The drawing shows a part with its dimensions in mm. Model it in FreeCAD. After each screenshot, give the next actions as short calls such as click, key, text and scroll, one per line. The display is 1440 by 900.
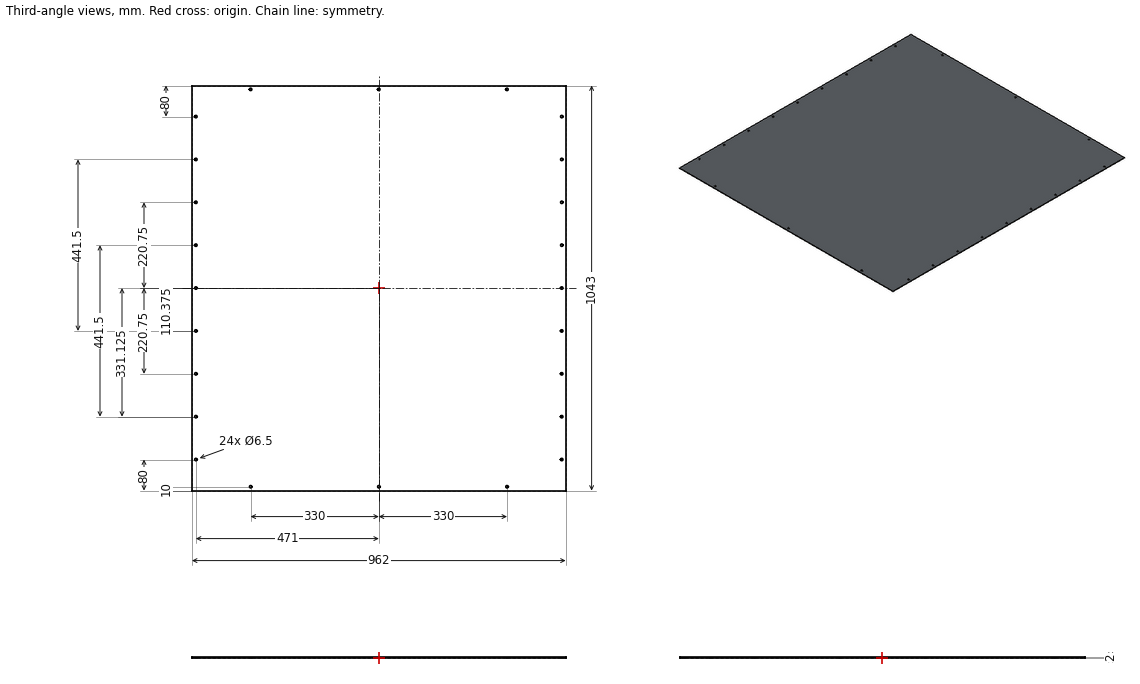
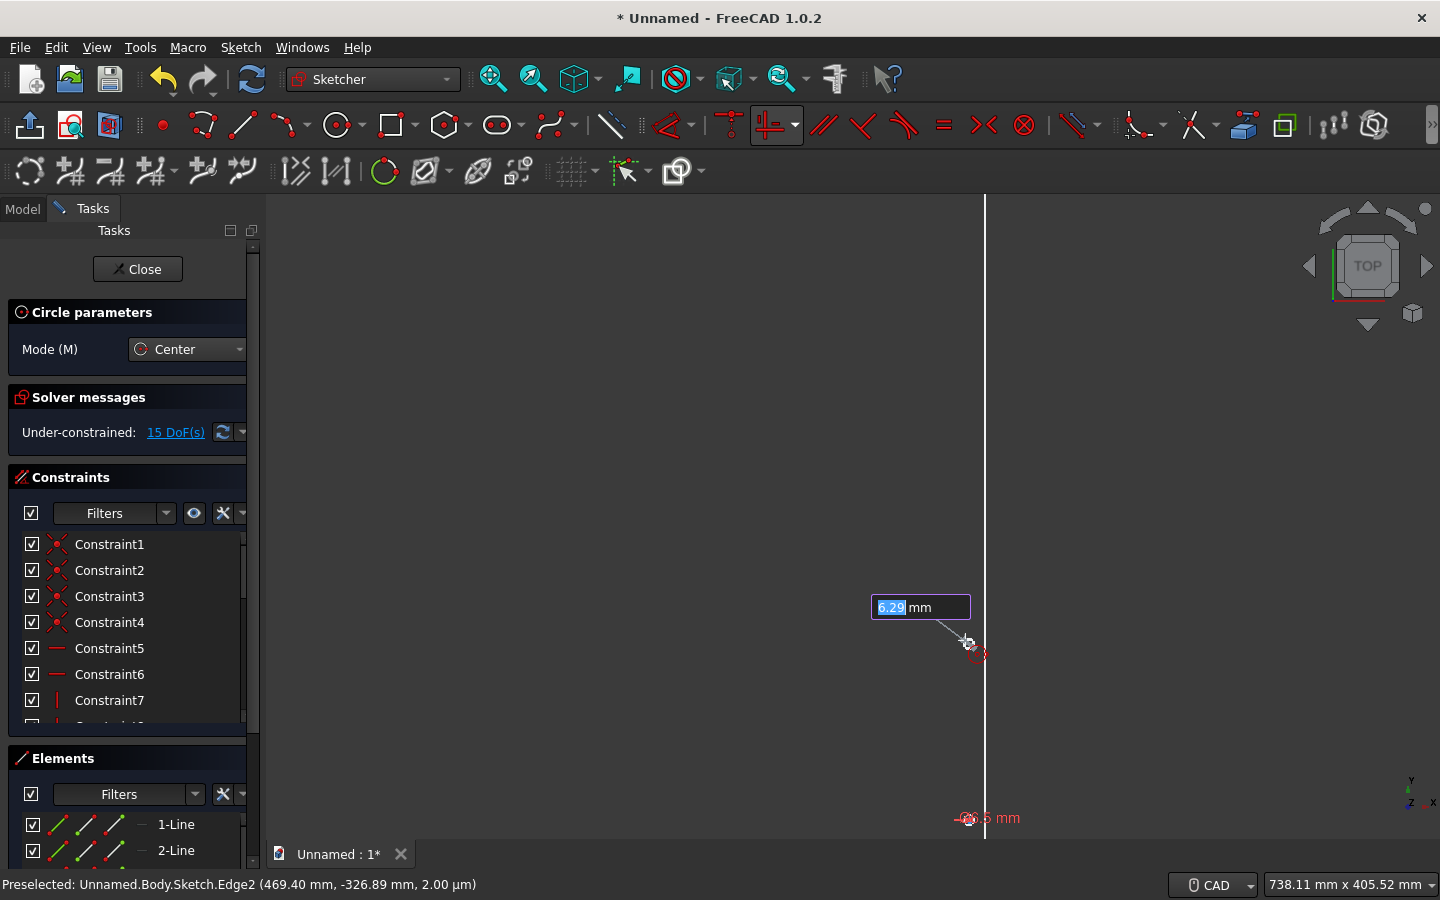
text(6.5)
key(Return)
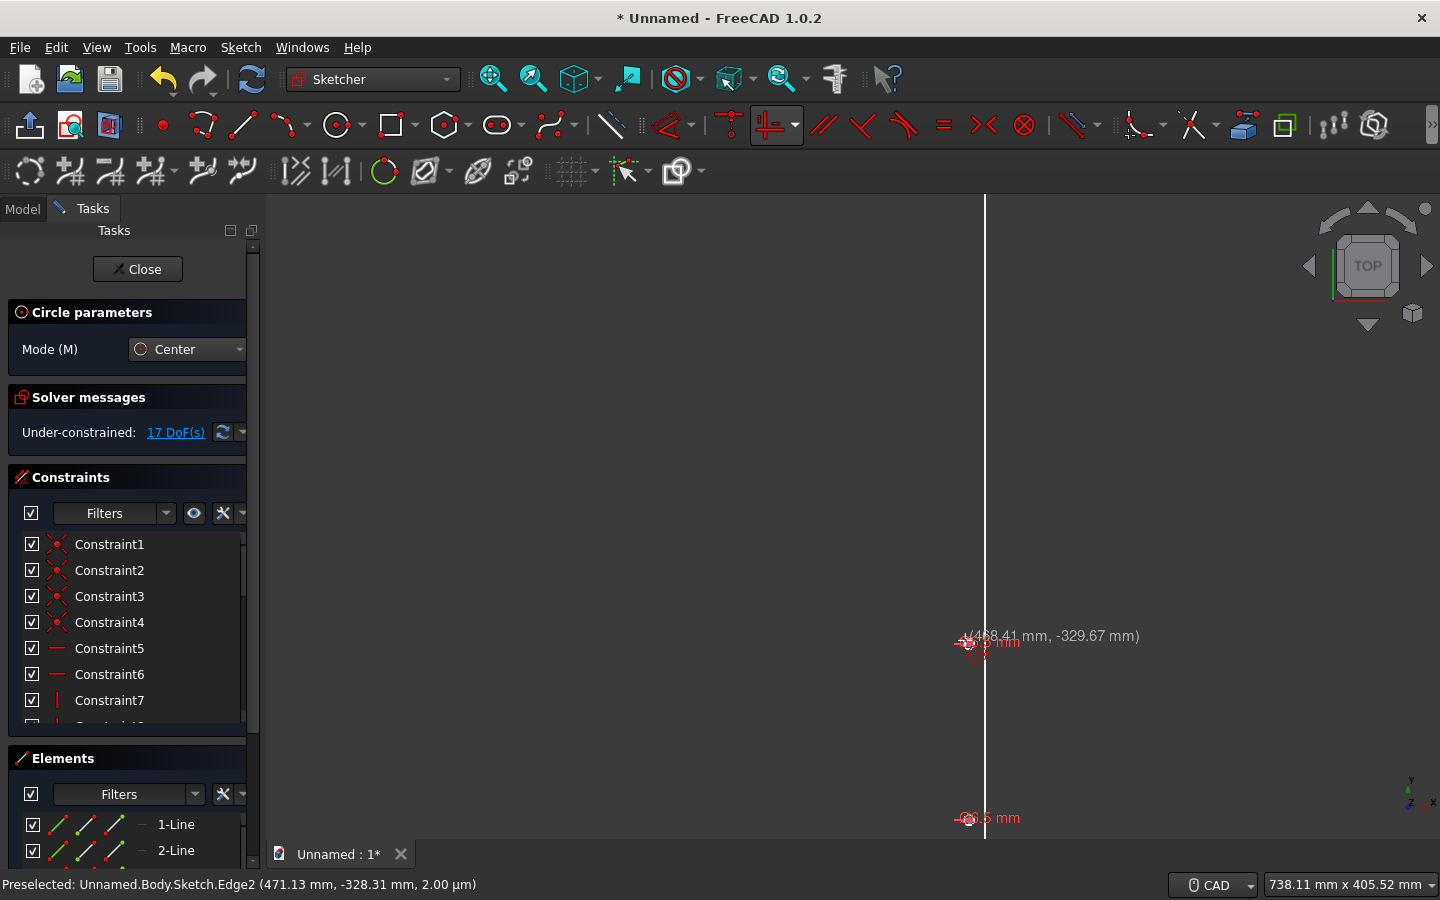
scroll(969, 468, up, 8)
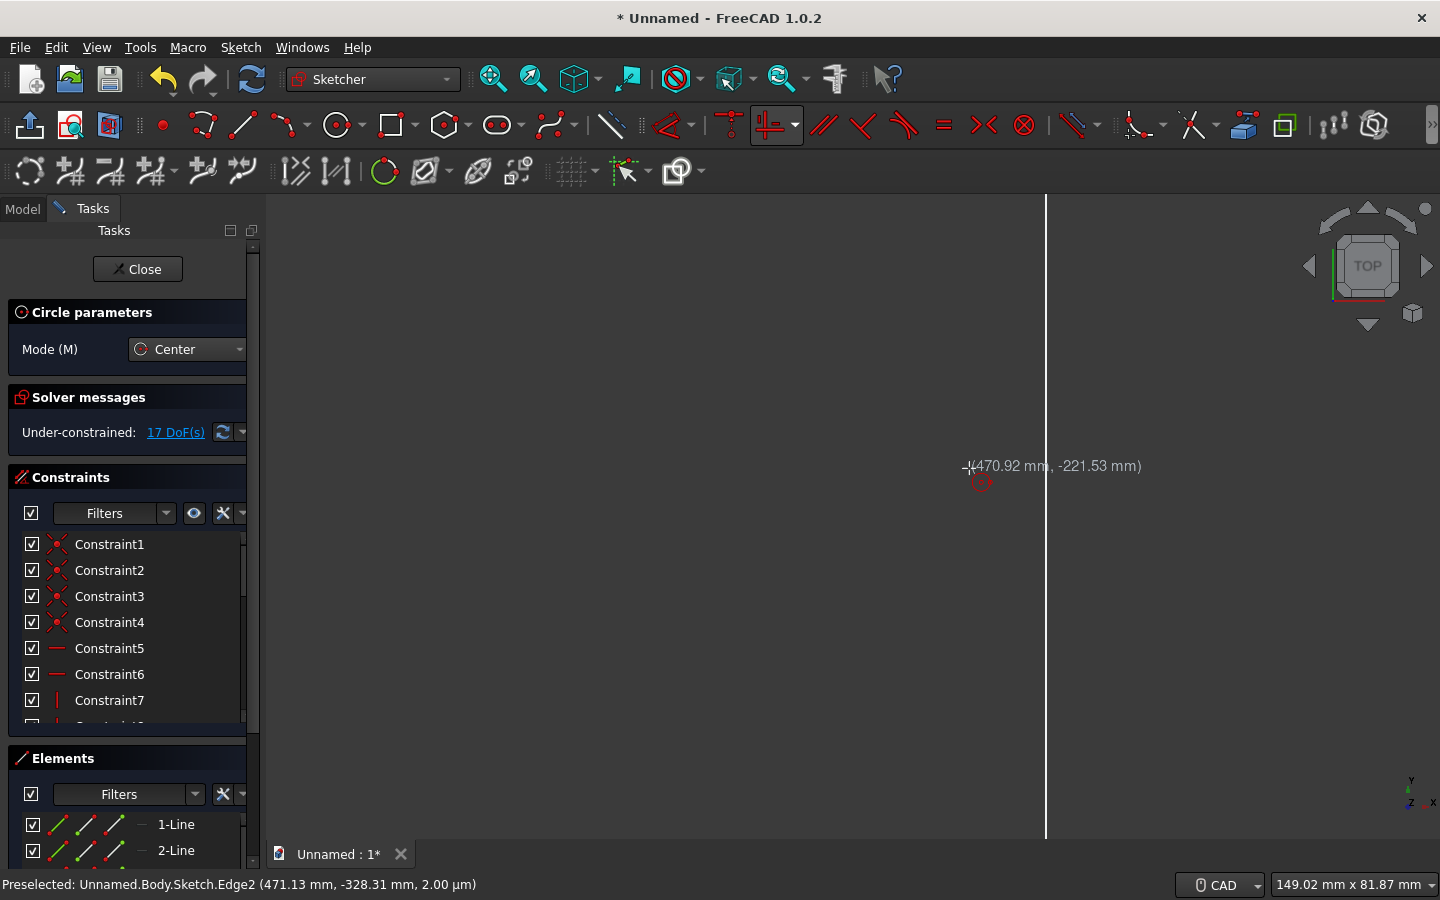
scroll(969, 610, down, 15)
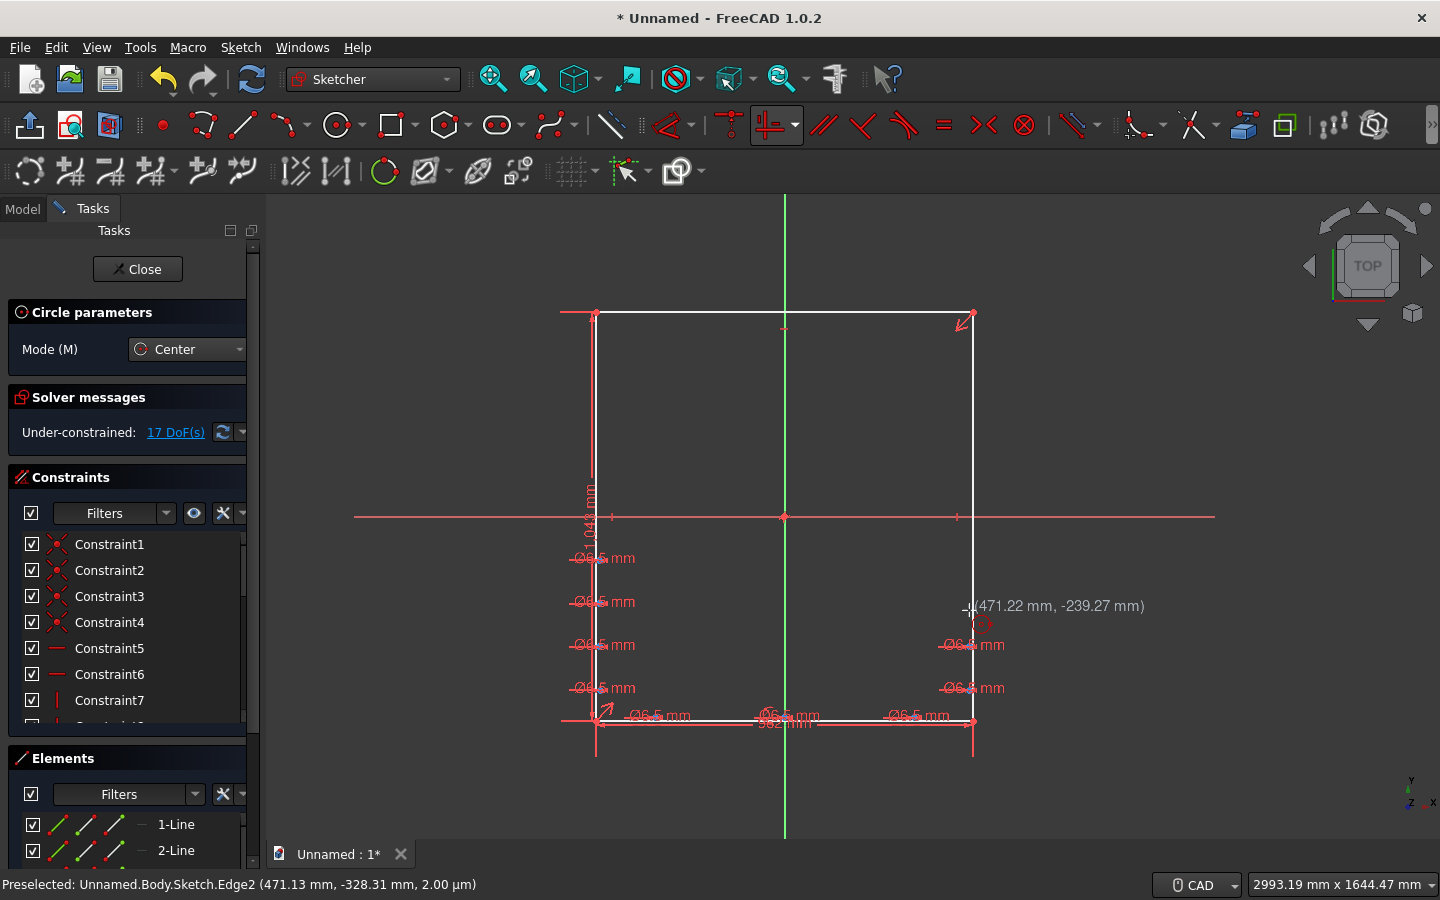
scroll(969, 603, up, 7)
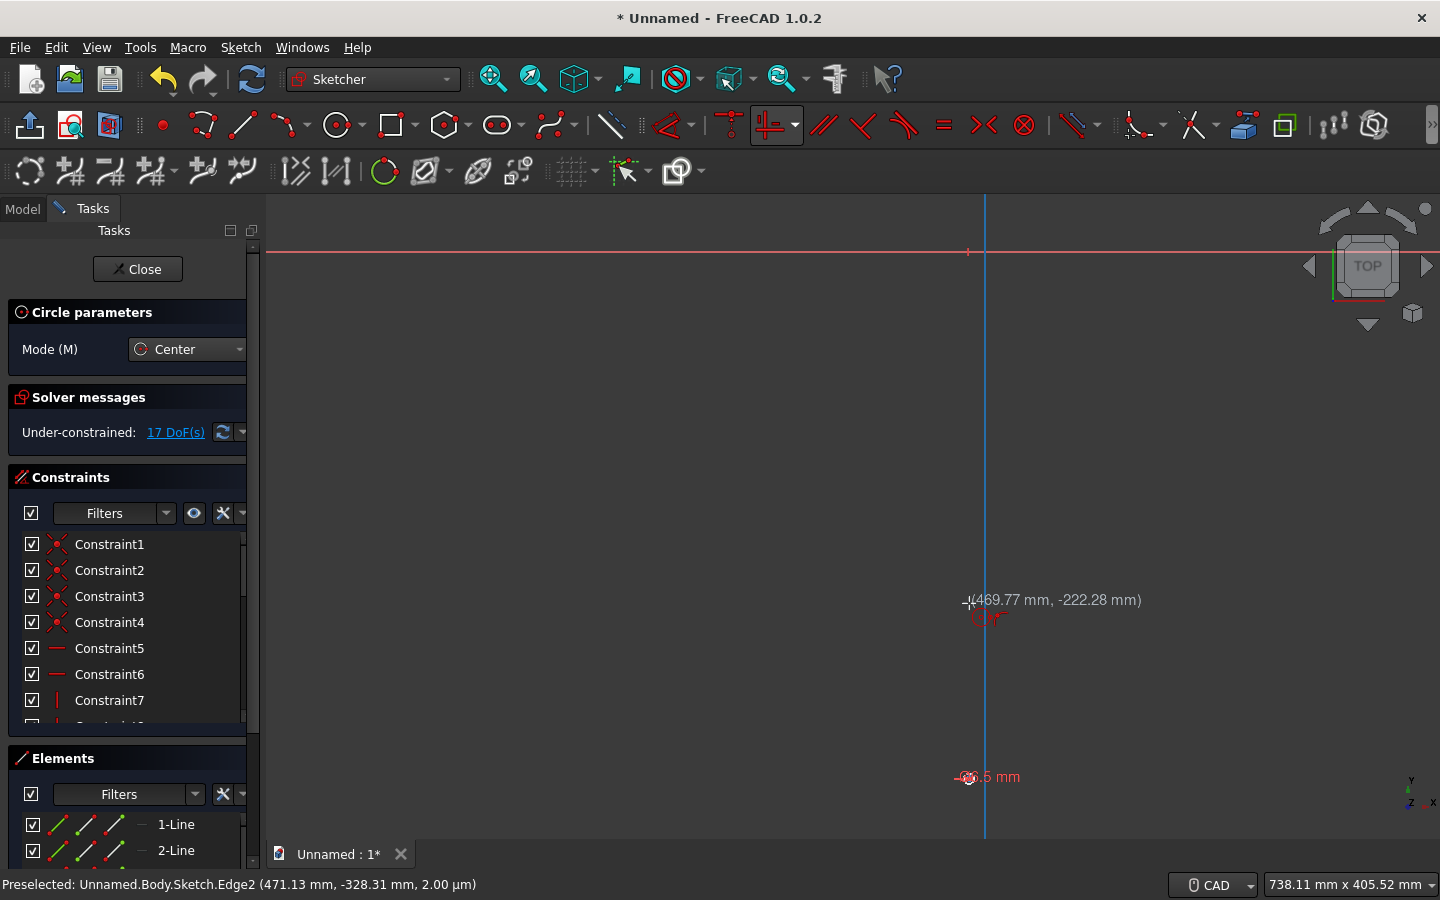
click(969, 603)
move(965, 599)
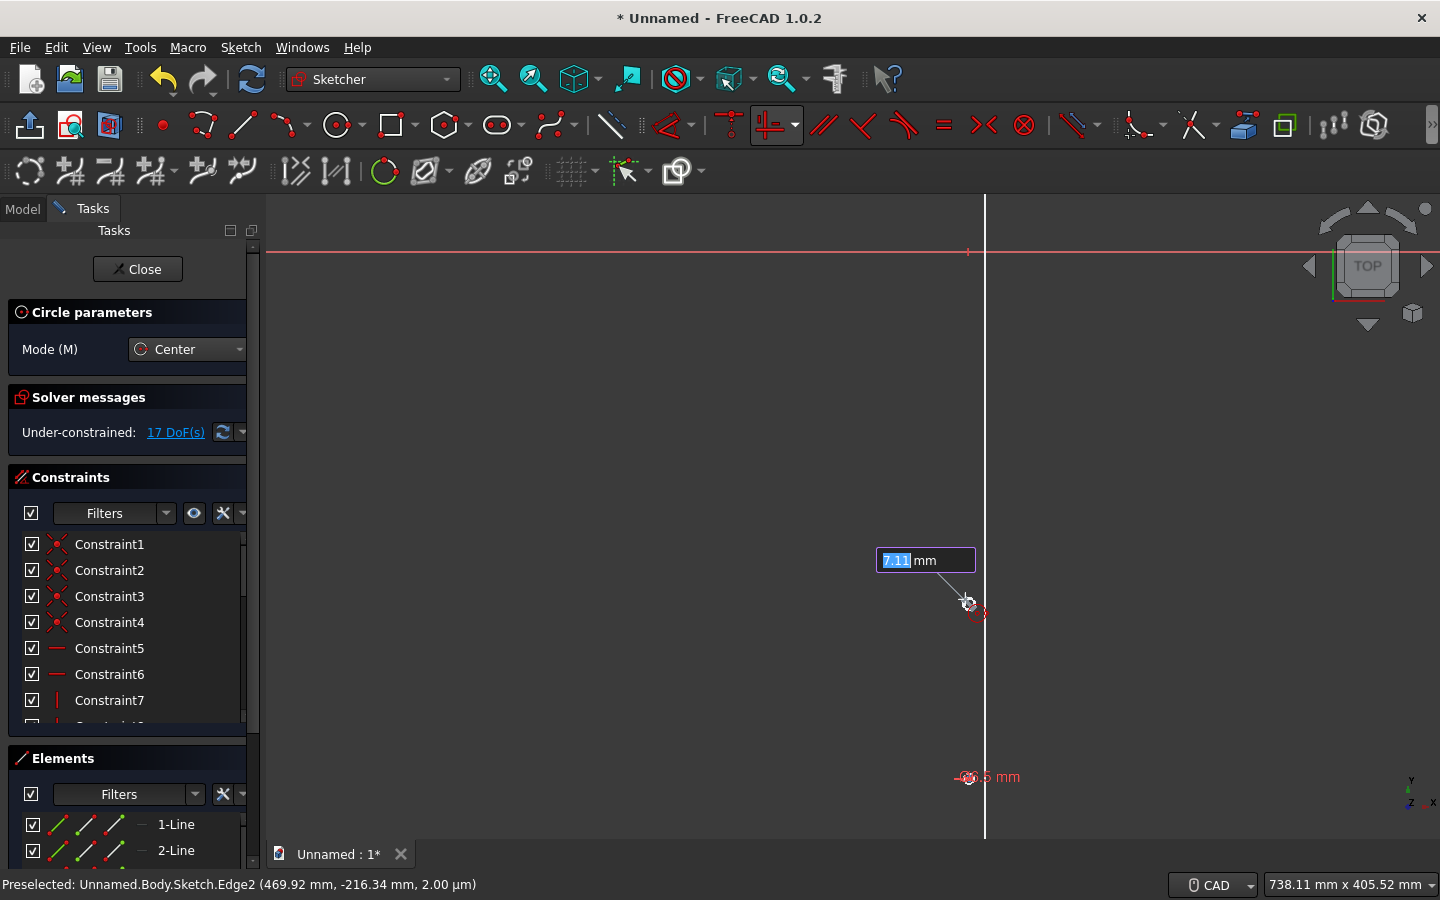
text(6.5)
key(Return)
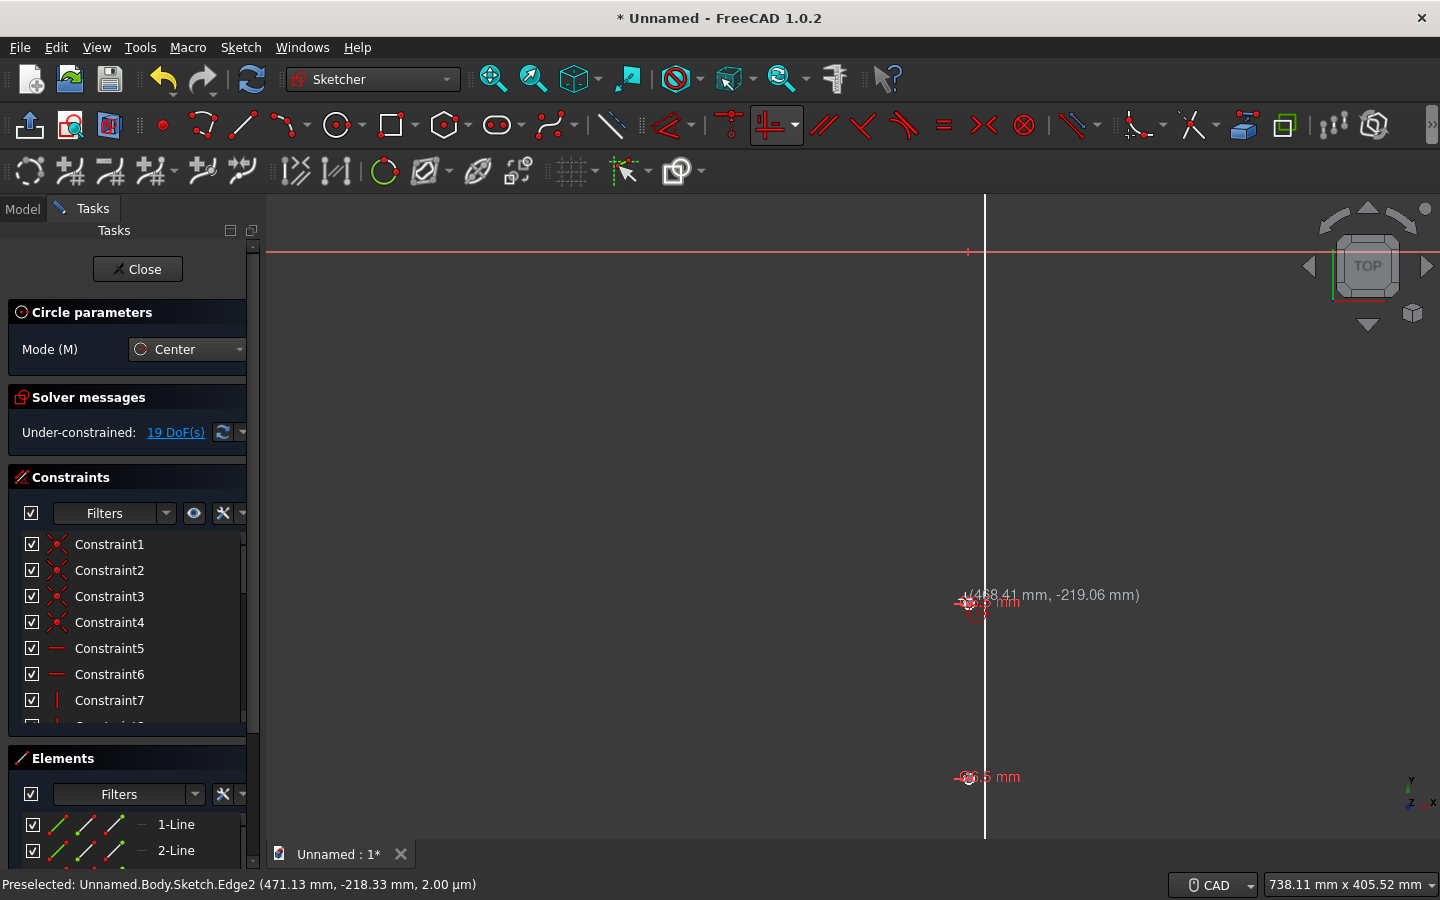
scroll(969, 427, up, 8)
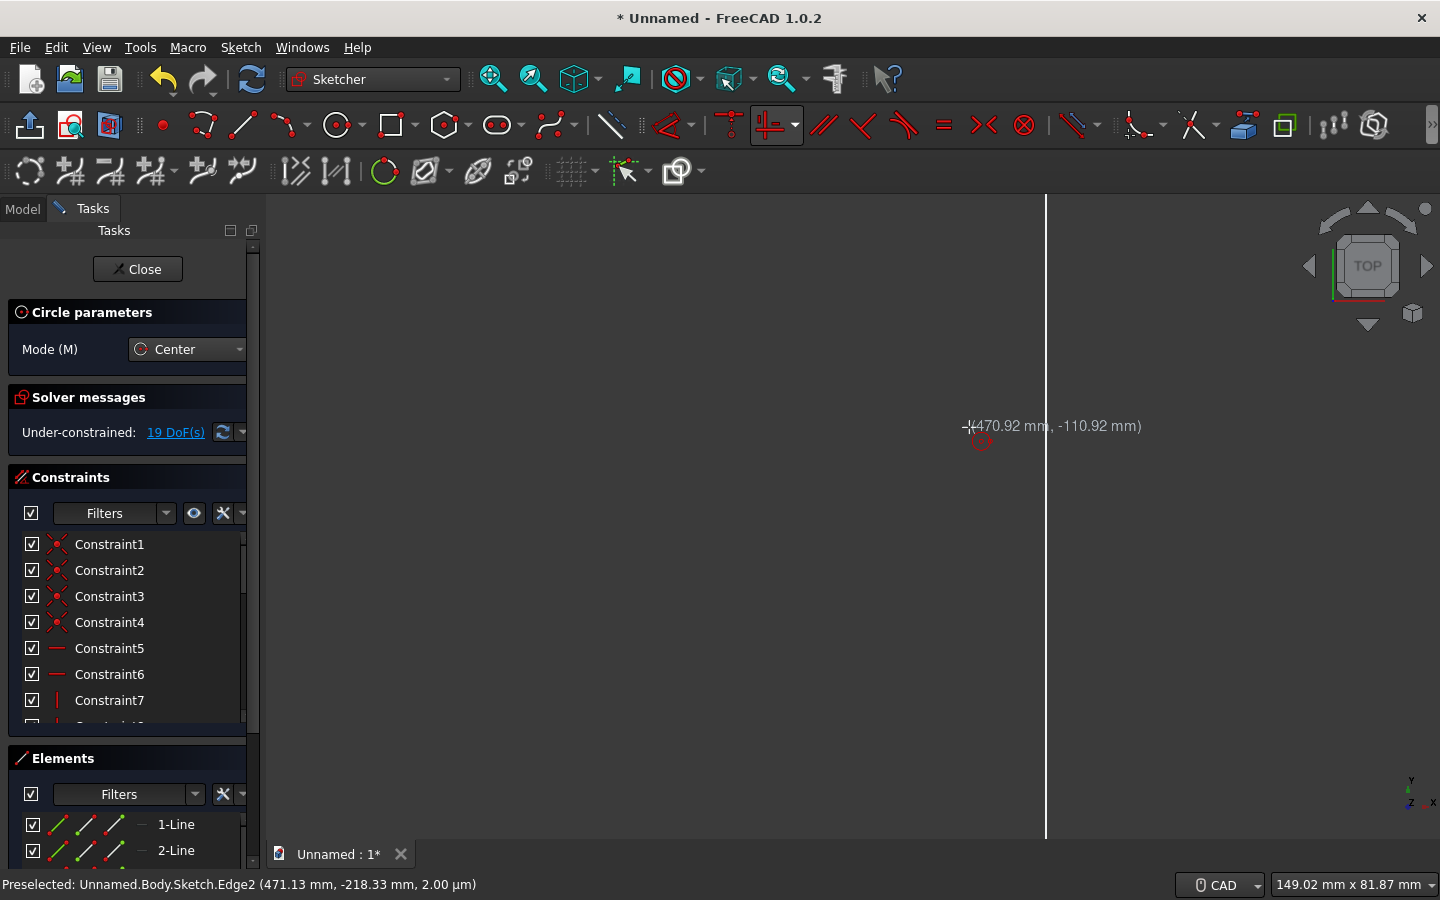
scroll(969, 567, down, 15)